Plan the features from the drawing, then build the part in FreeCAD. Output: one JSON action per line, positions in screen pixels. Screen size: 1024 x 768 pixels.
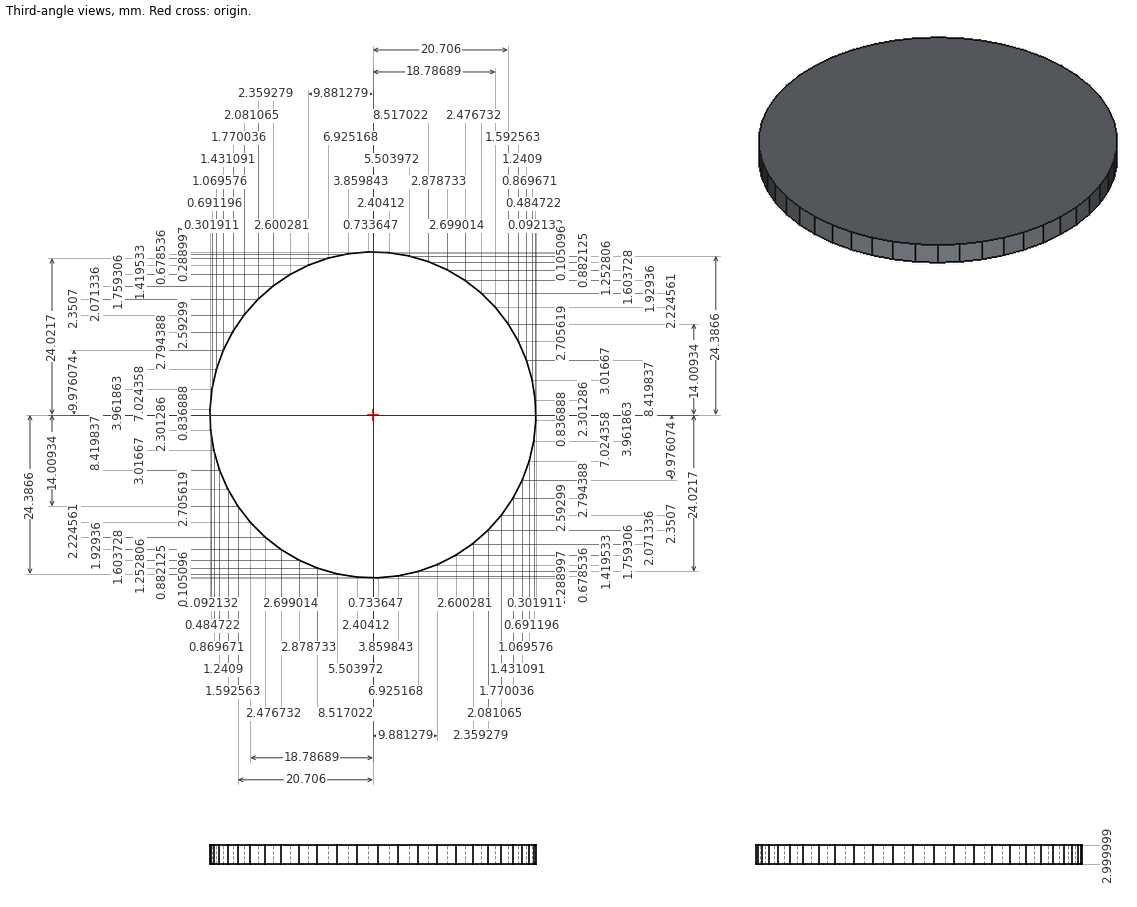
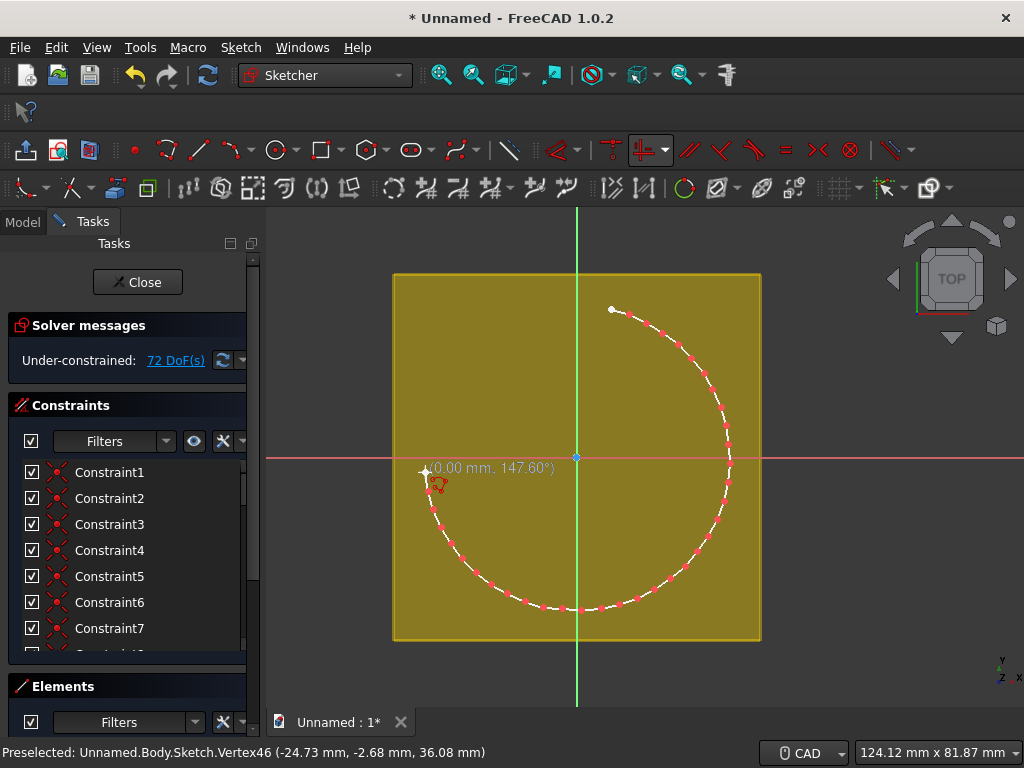
{"action": "scroll", "coordinate": [424, 452], "scroll_direction": "up", "scroll_amount": 6}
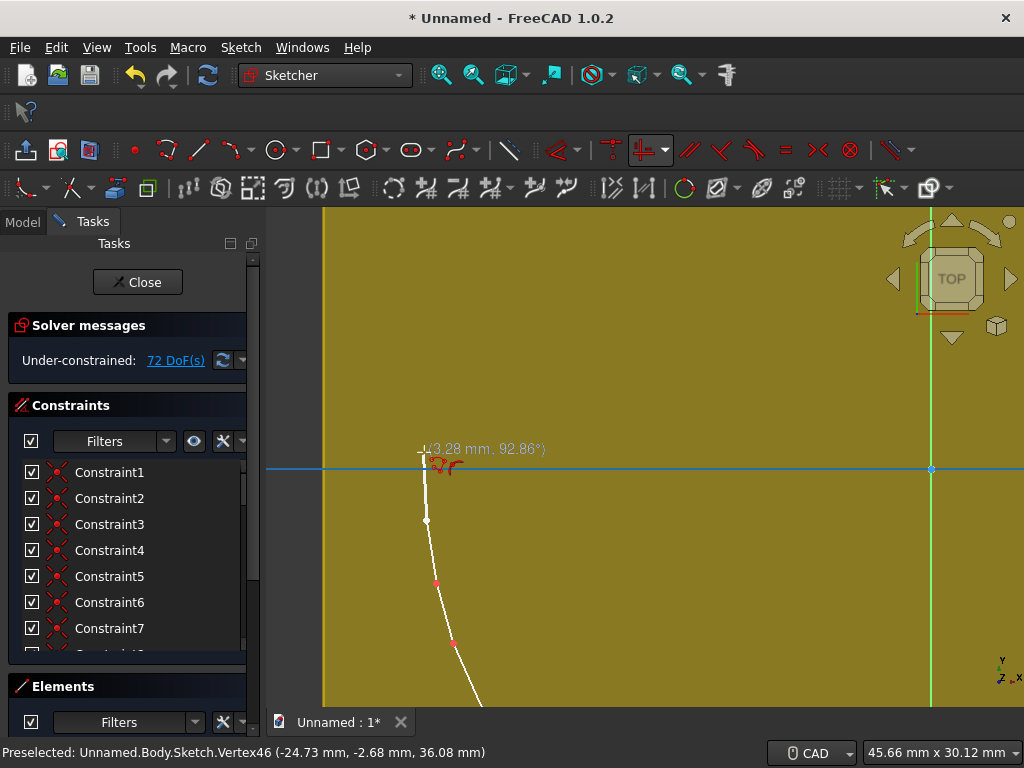
{"action": "left_click", "coordinate": [422, 453]}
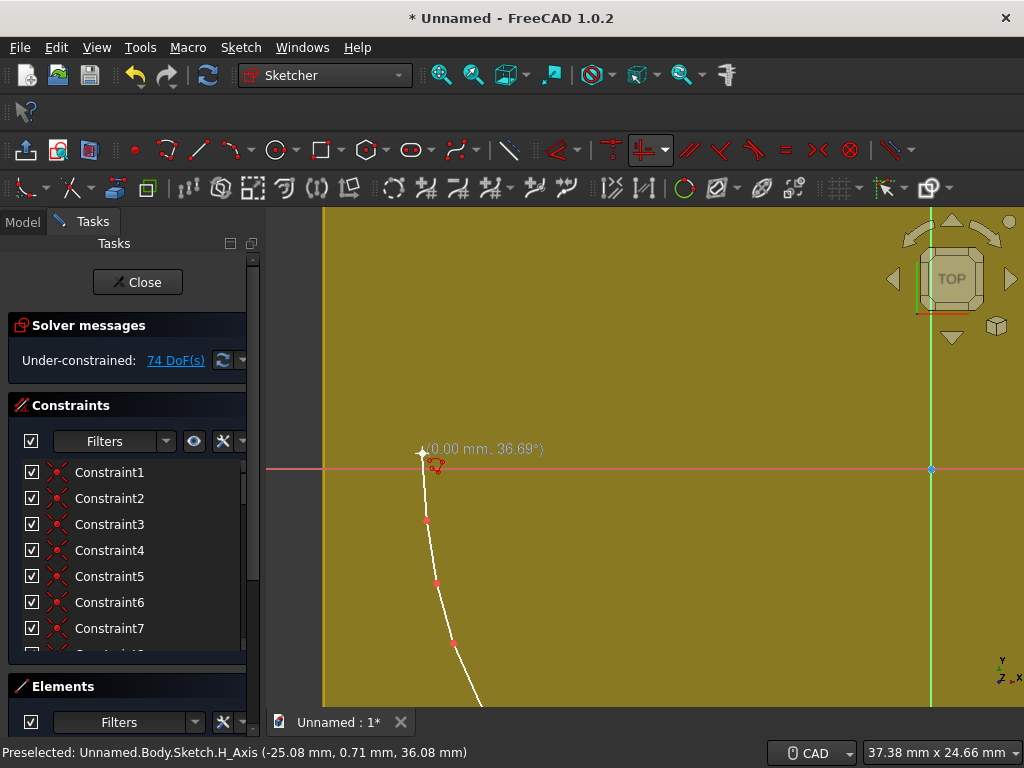
{"action": "scroll", "coordinate": [423, 452], "scroll_direction": "down", "scroll_amount": 6}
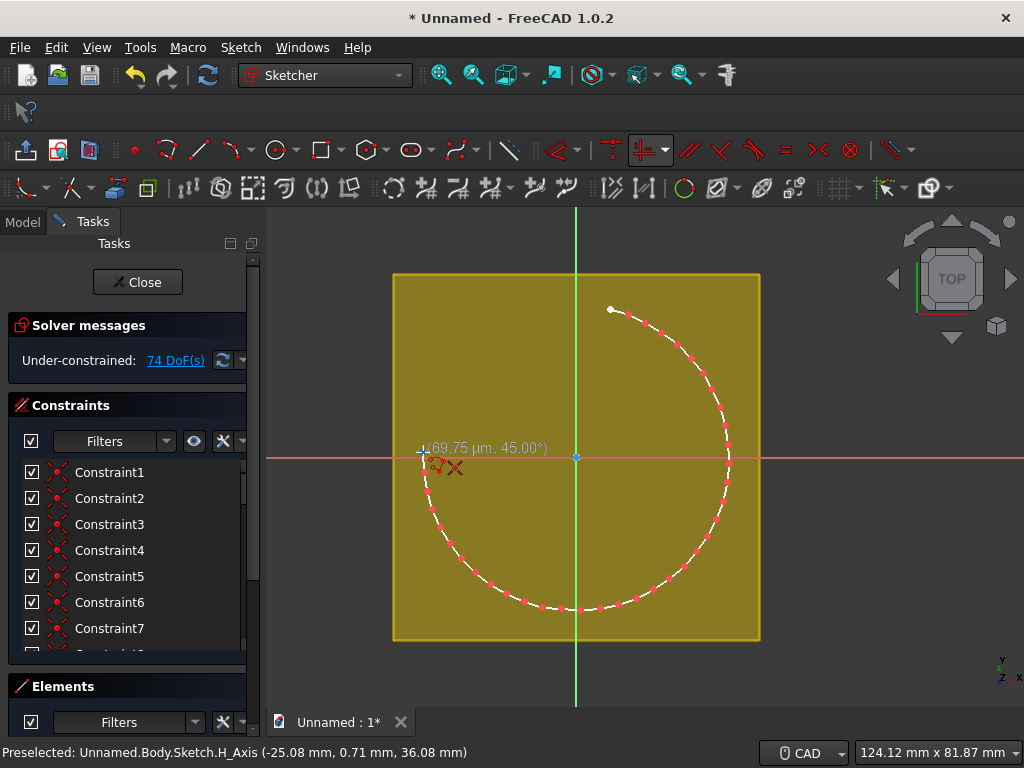
{"action": "left_click", "coordinate": [425, 433]}
{"action": "left_click", "coordinate": [430, 415]}
{"action": "left_click", "coordinate": [436, 397]}
{"action": "left_click", "coordinate": [445, 380]}
{"action": "left_click", "coordinate": [456, 364]}
{"action": "left_click", "coordinate": [469, 349]}
{"action": "left_click", "coordinate": [483, 337]}
{"action": "left_click", "coordinate": [499, 326]}
{"action": "left_click", "coordinate": [516, 317]}
{"action": "left_click", "coordinate": [534, 311]}
{"action": "left_click", "coordinate": [553, 307]}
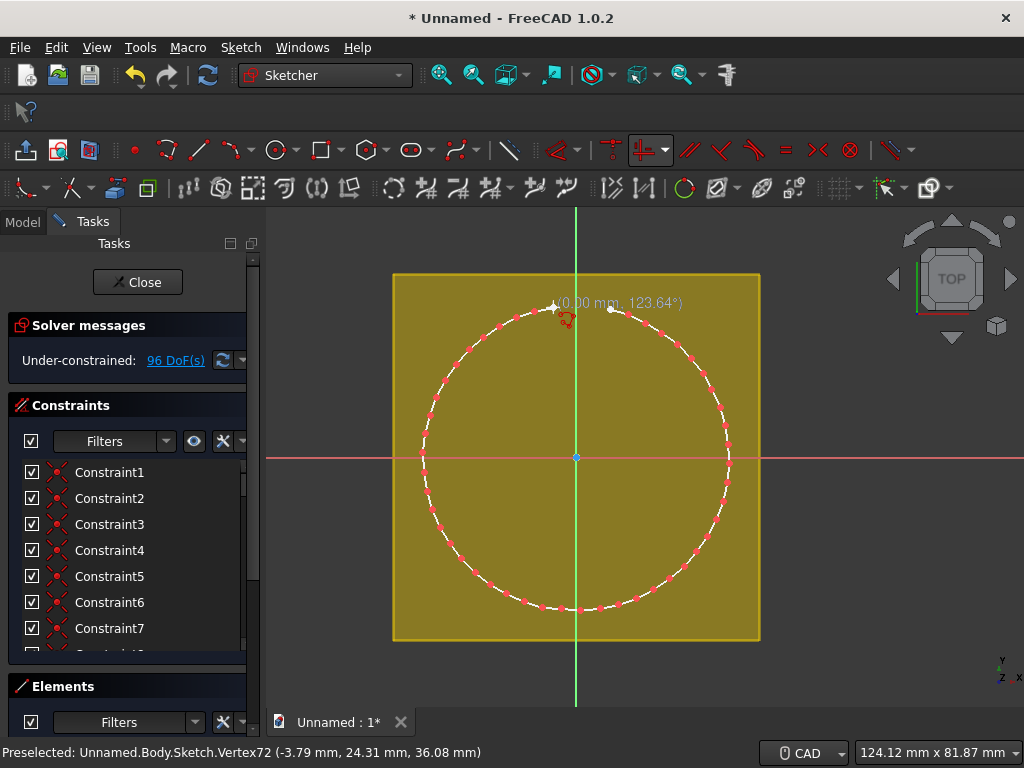
{"action": "scroll", "coordinate": [572, 305], "scroll_direction": "up", "scroll_amount": 7}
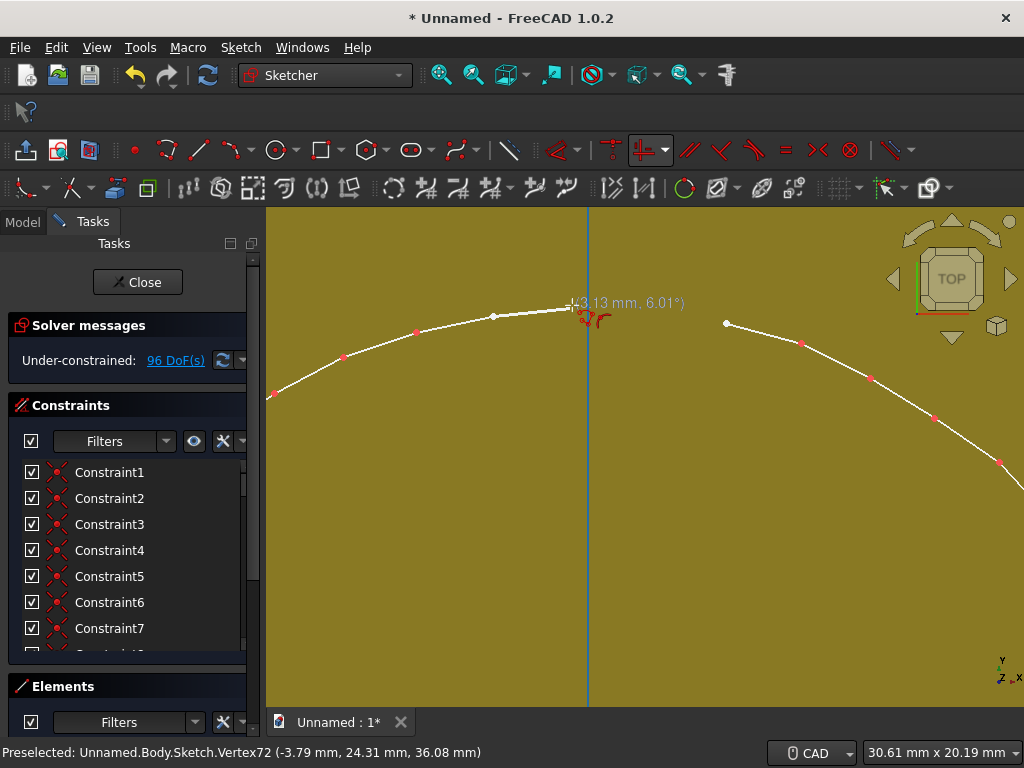
{"action": "left_click", "coordinate": [570, 304]}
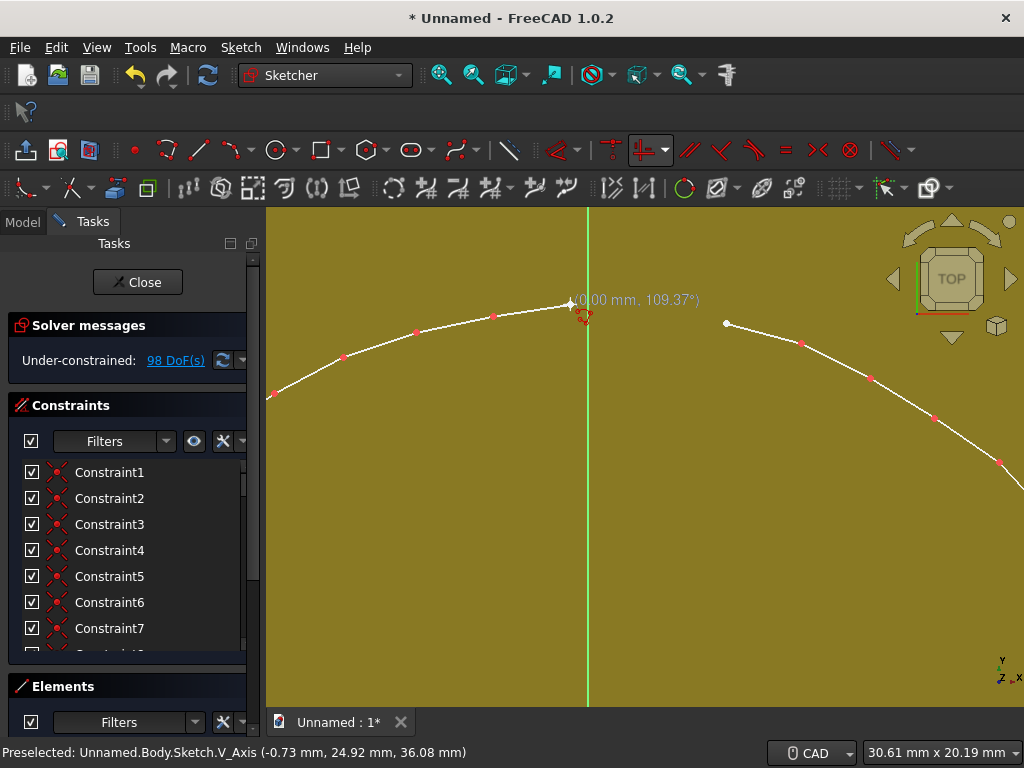
{"action": "scroll", "coordinate": [573, 304], "scroll_direction": "down", "scroll_amount": 7}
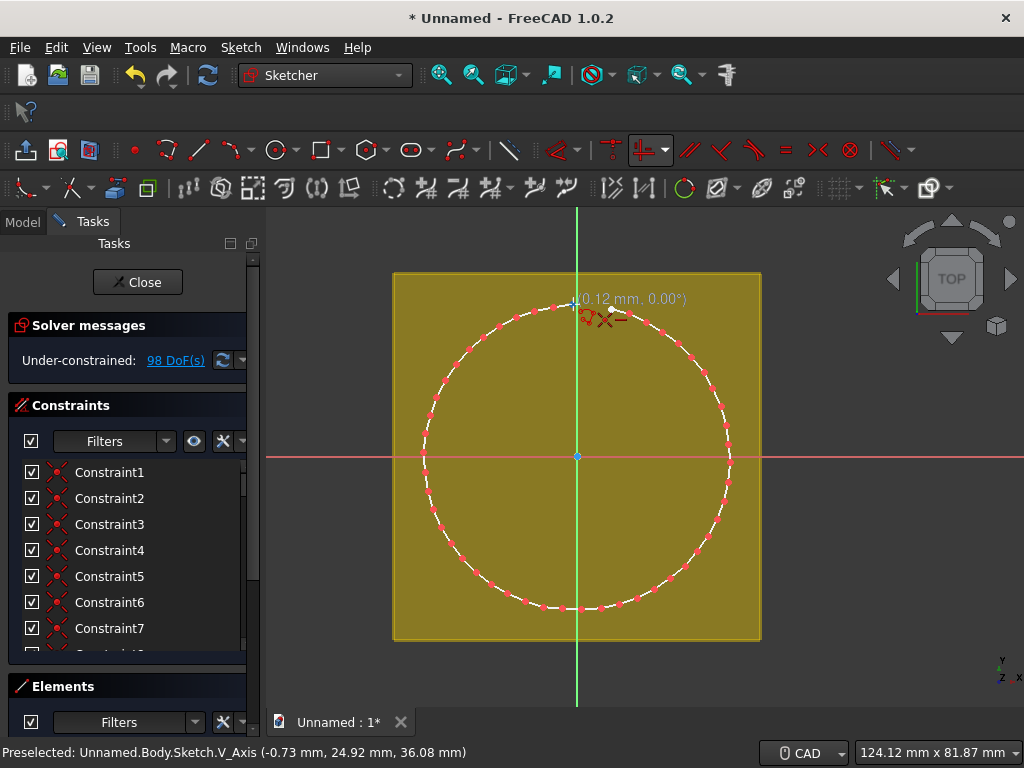
{"action": "left_click", "coordinate": [592, 307]}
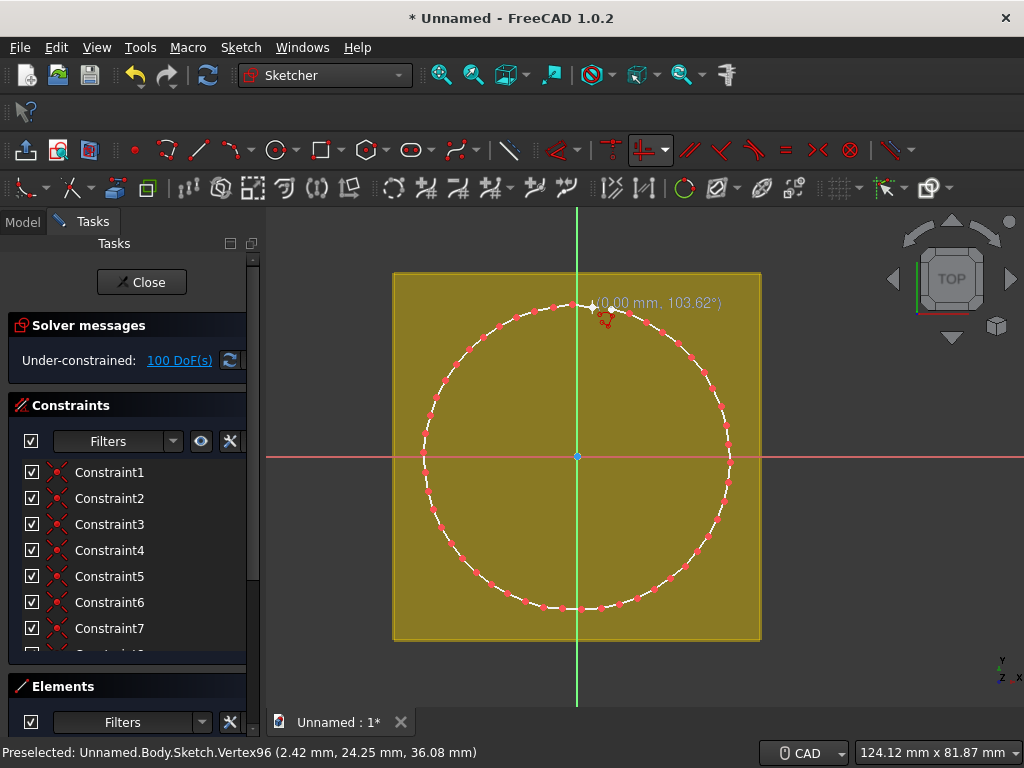
{"action": "scroll", "coordinate": [611, 308], "scroll_direction": "up", "scroll_amount": 3}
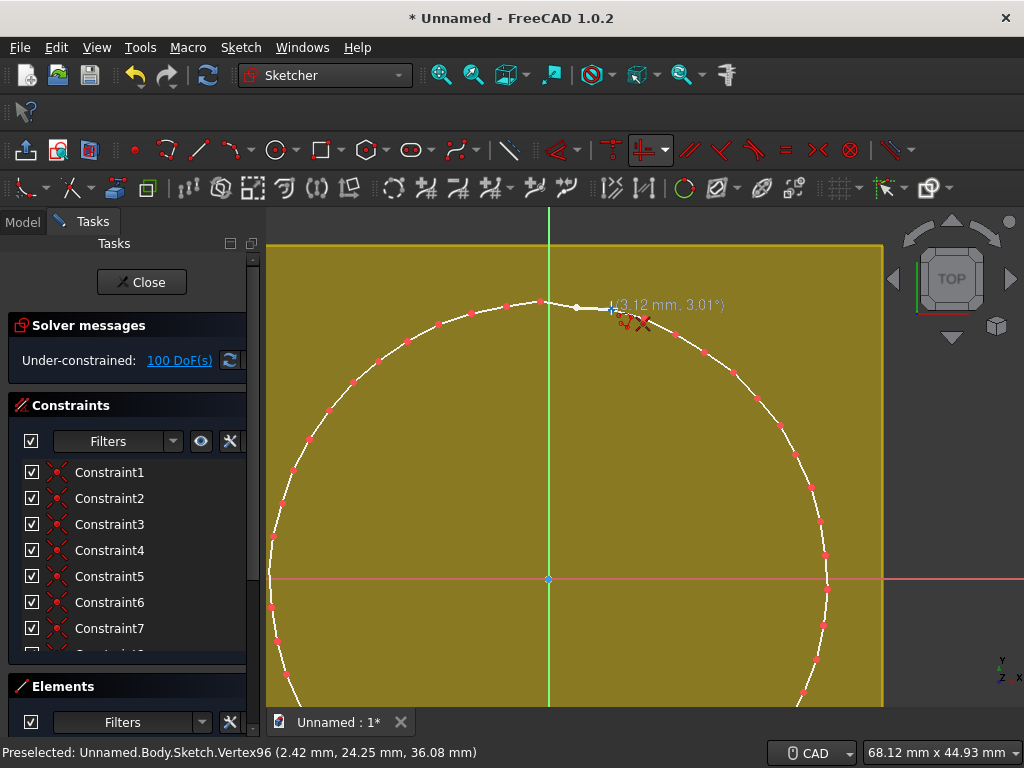
{"action": "left_click", "coordinate": [611, 310]}
{"action": "key", "text": "Escape"}
{"action": "key", "text": "Escape"}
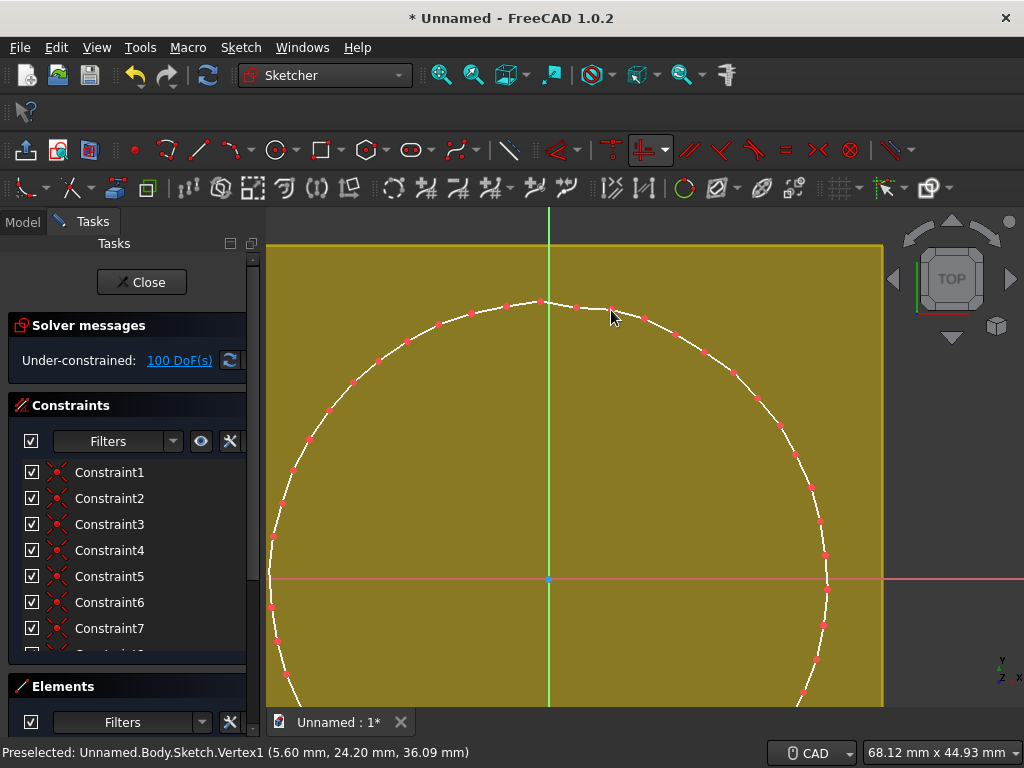
{"action": "left_click", "coordinate": [556, 150]}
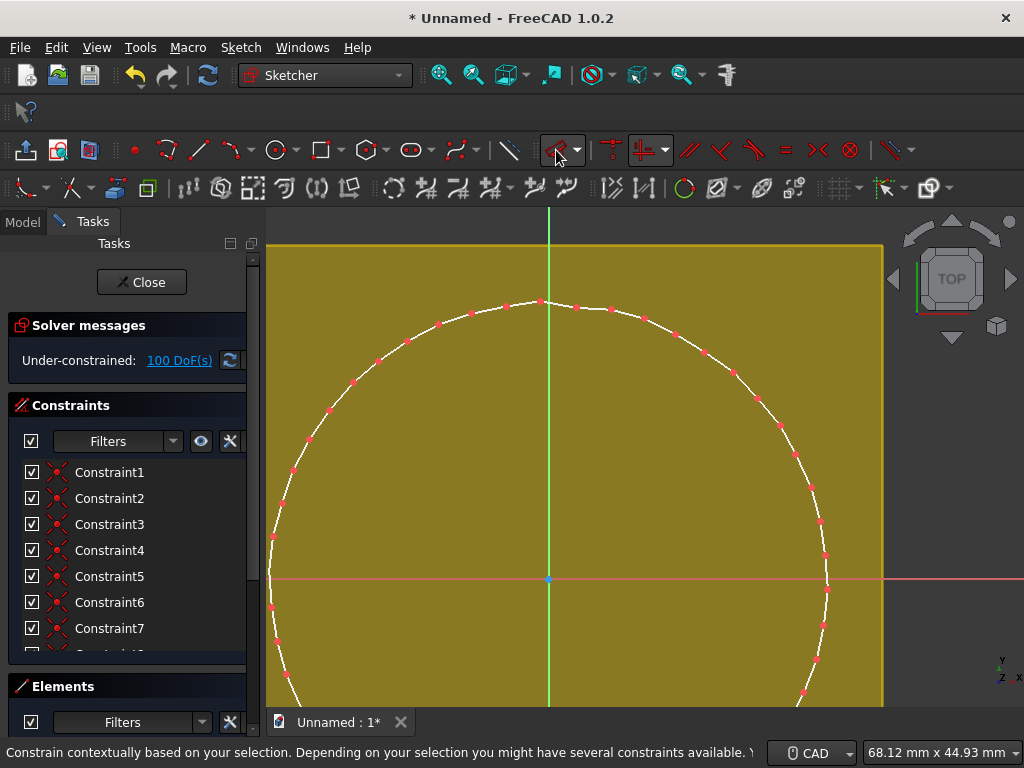
{"action": "left_click", "coordinate": [780, 426]}
{"action": "left_click", "coordinate": [664, 392]}